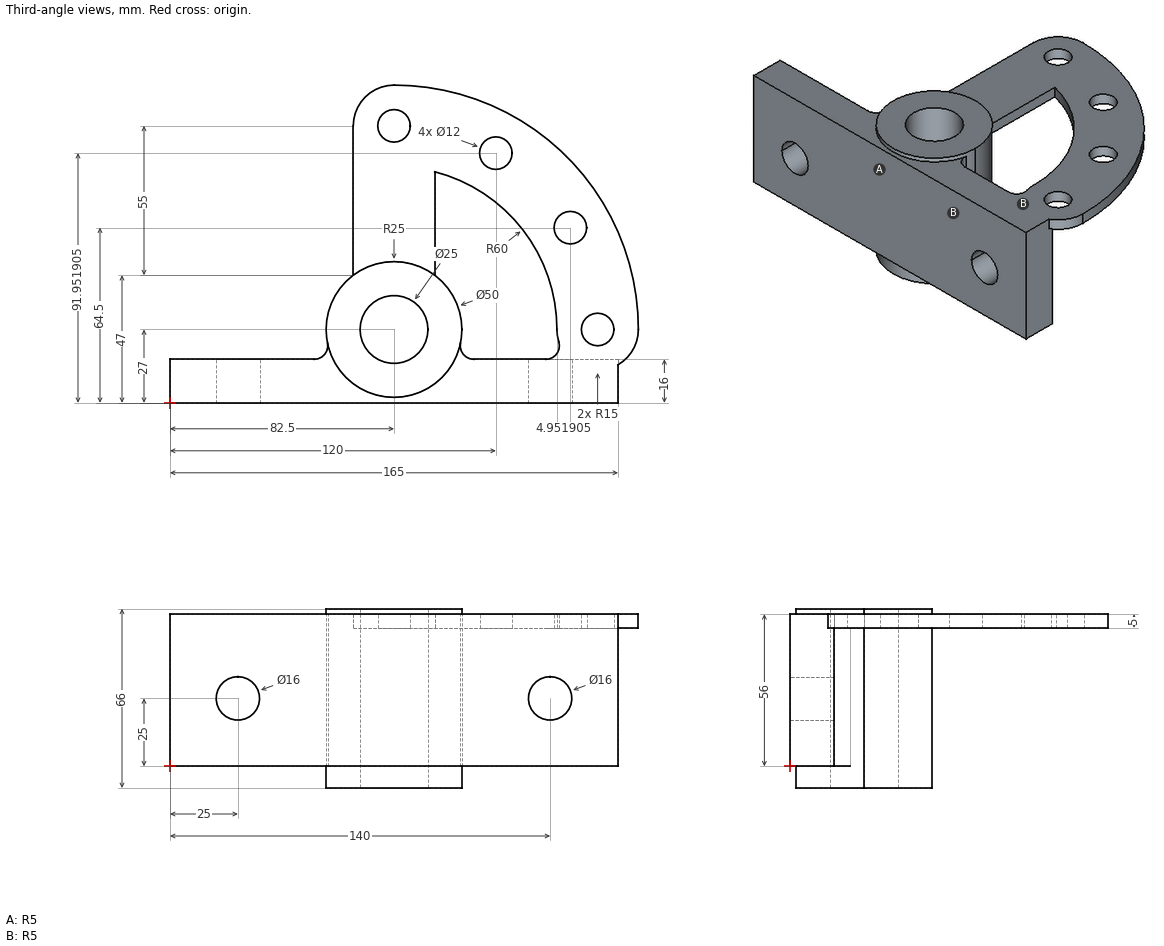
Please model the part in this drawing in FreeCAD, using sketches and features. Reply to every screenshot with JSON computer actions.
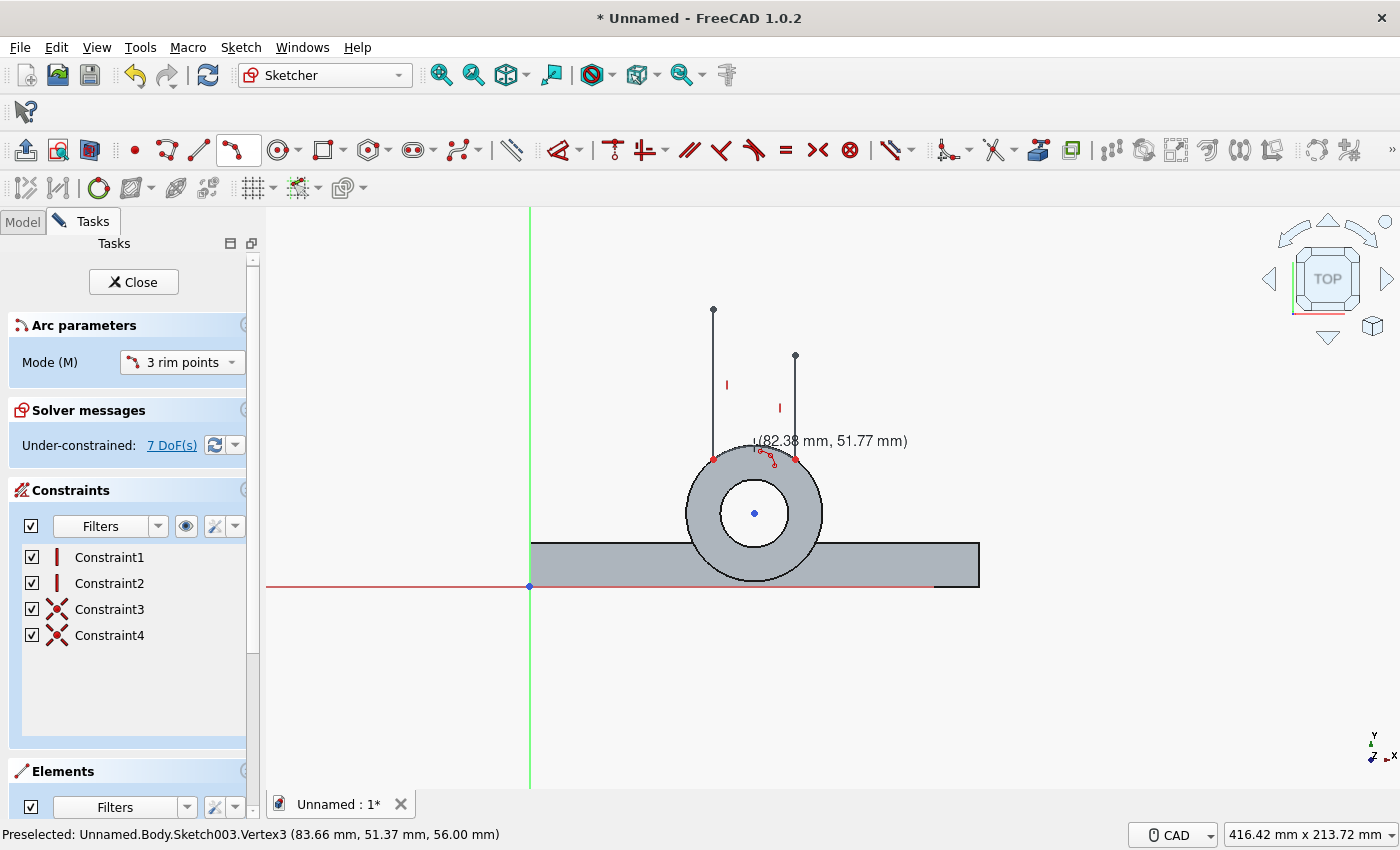
{"action": "left_click", "coordinate": [795, 356]}
{"action": "left_click", "coordinate": [918, 513]}
{"action": "left_click", "coordinate": [884, 413]}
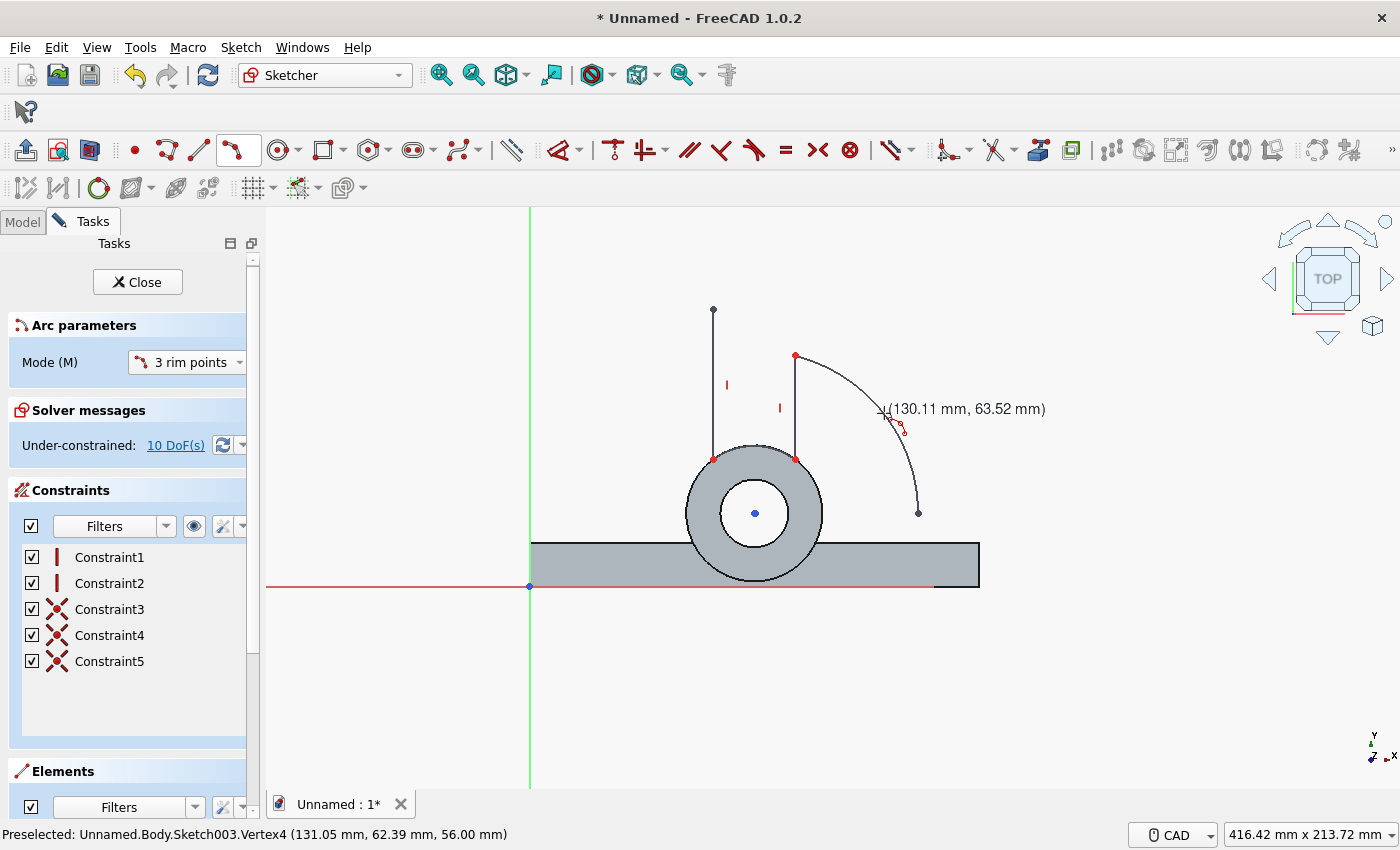
{"action": "left_click", "coordinate": [918, 514]}
{"action": "left_click", "coordinate": [999, 513]}
{"action": "left_click", "coordinate": [959, 554]}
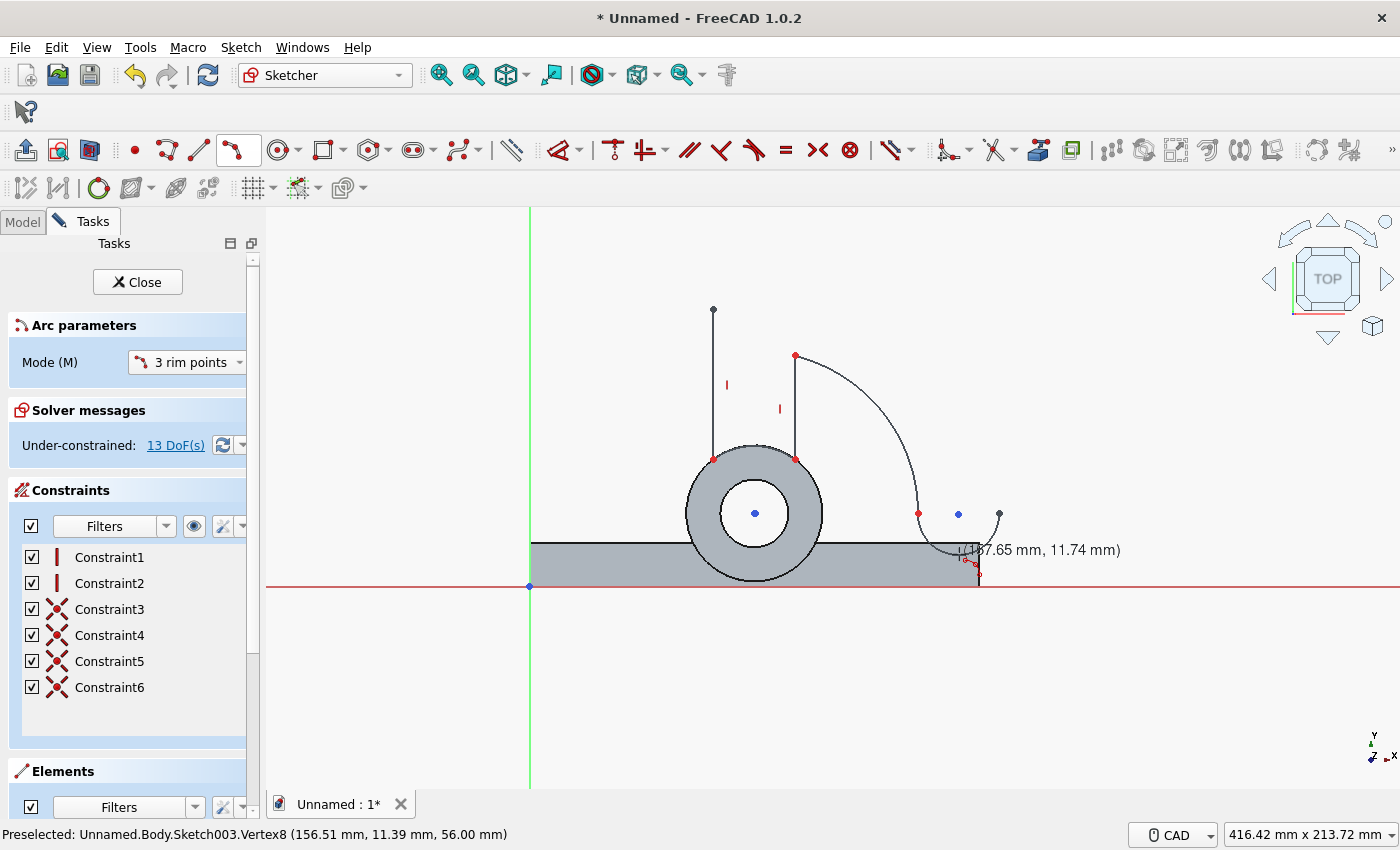
{"action": "left_click", "coordinate": [999, 514]}
{"action": "left_click", "coordinate": [754, 268]}
{"action": "left_click", "coordinate": [928, 340]}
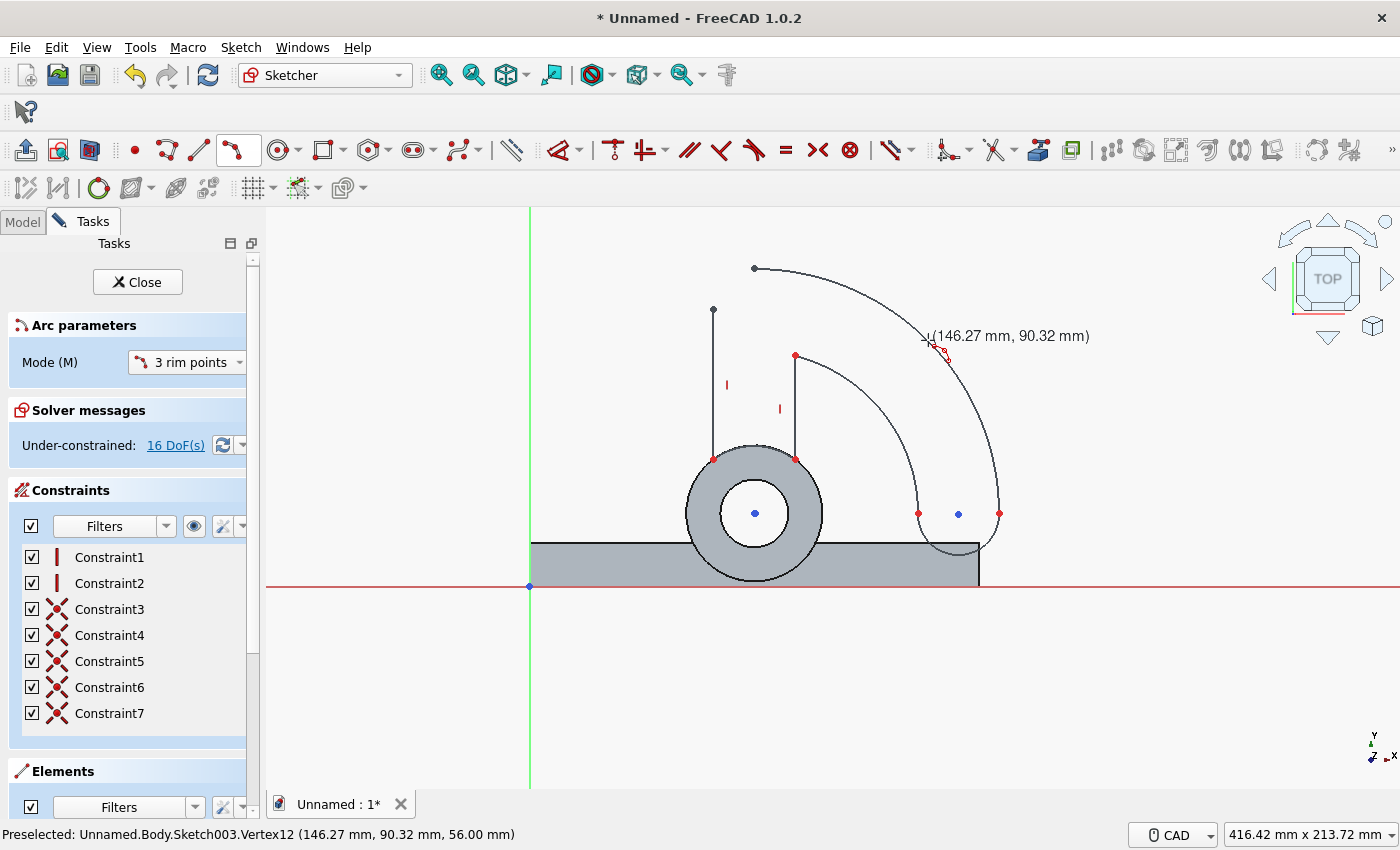
{"action": "left_click", "coordinate": [754, 269]}
{"action": "left_click", "coordinate": [713, 310]}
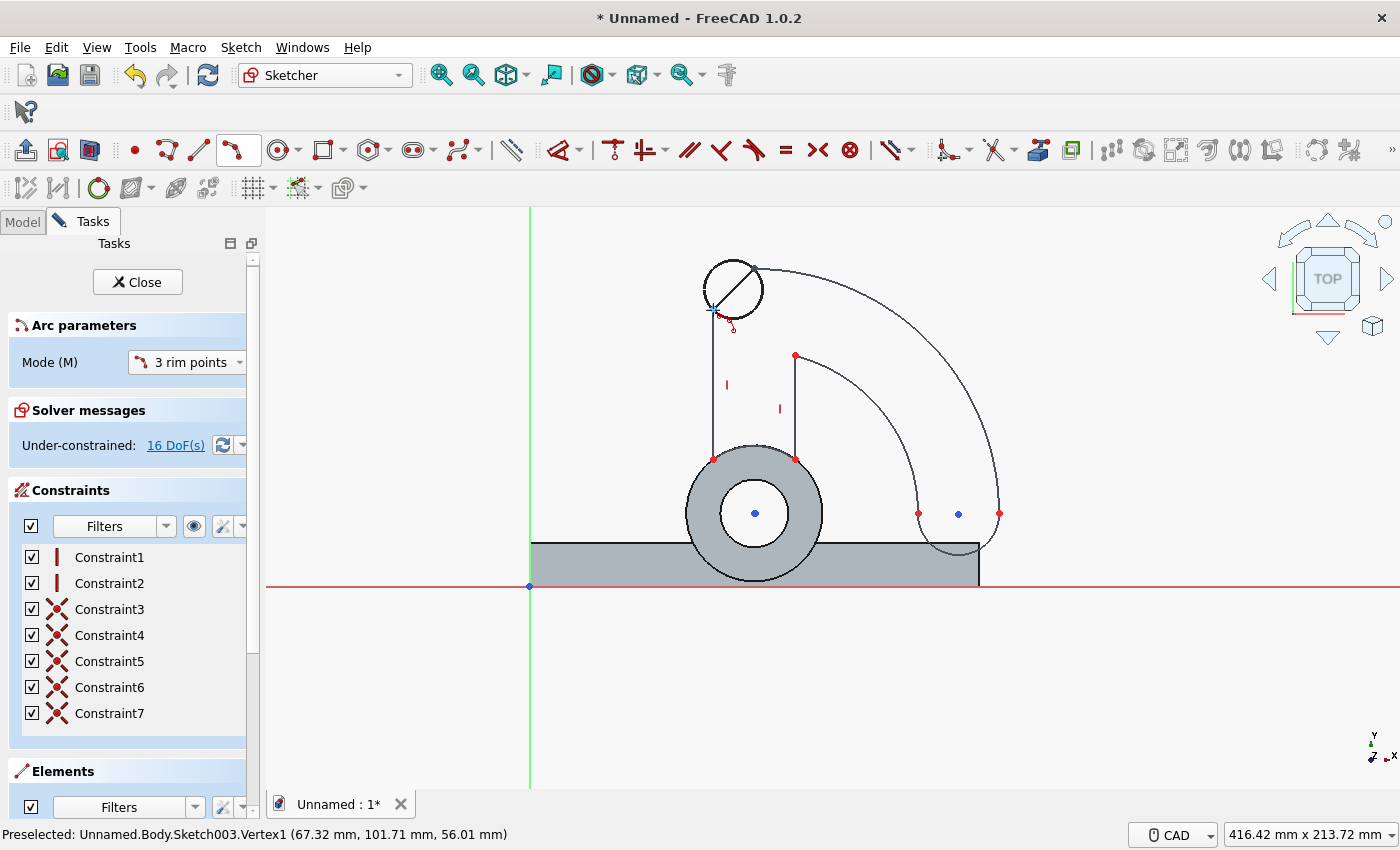
{"action": "scroll", "coordinate": [725, 280], "scroll_direction": "up", "scroll_amount": 2}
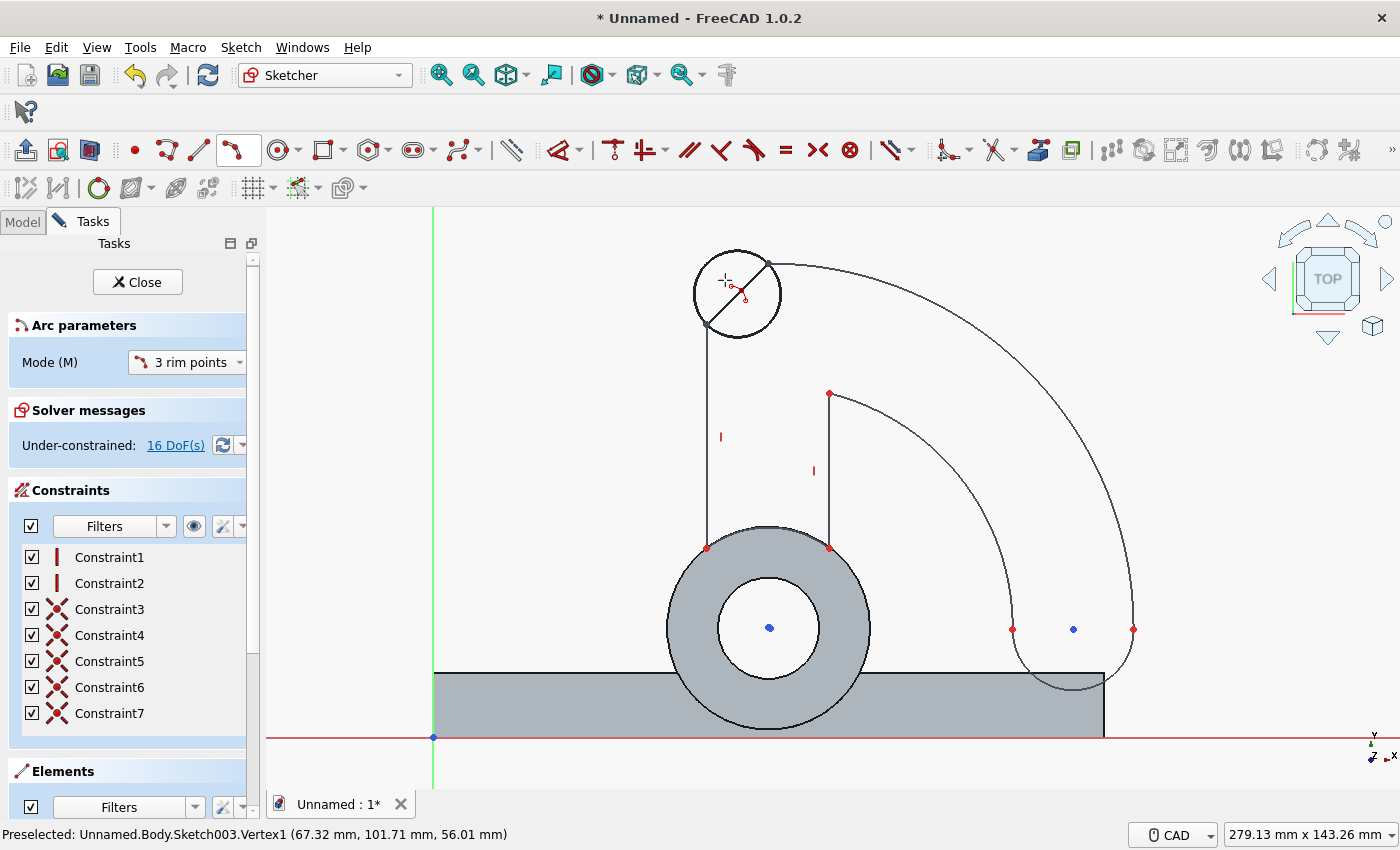
{"action": "left_click", "coordinate": [725, 280]}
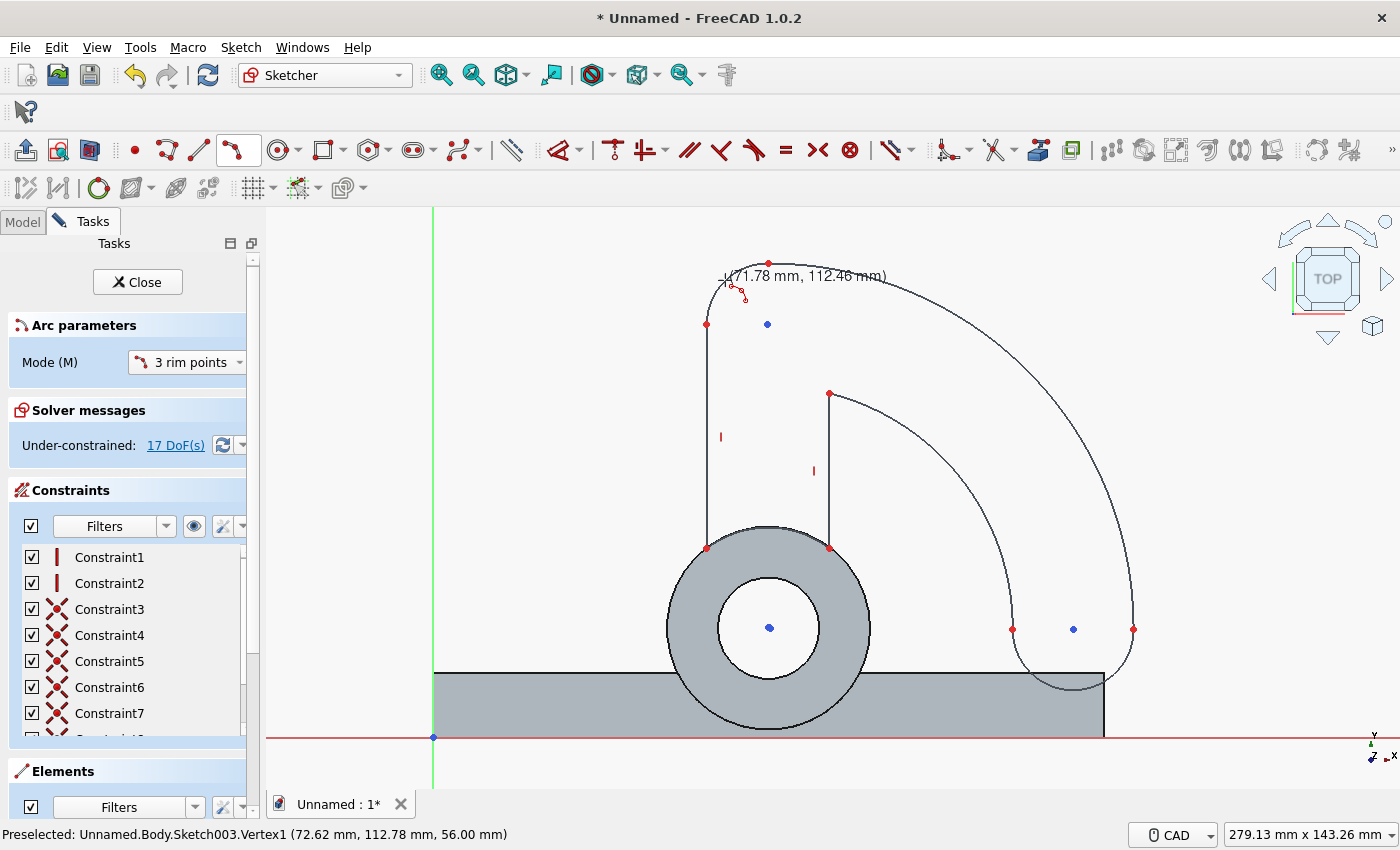
{"action": "key", "text": "g c"}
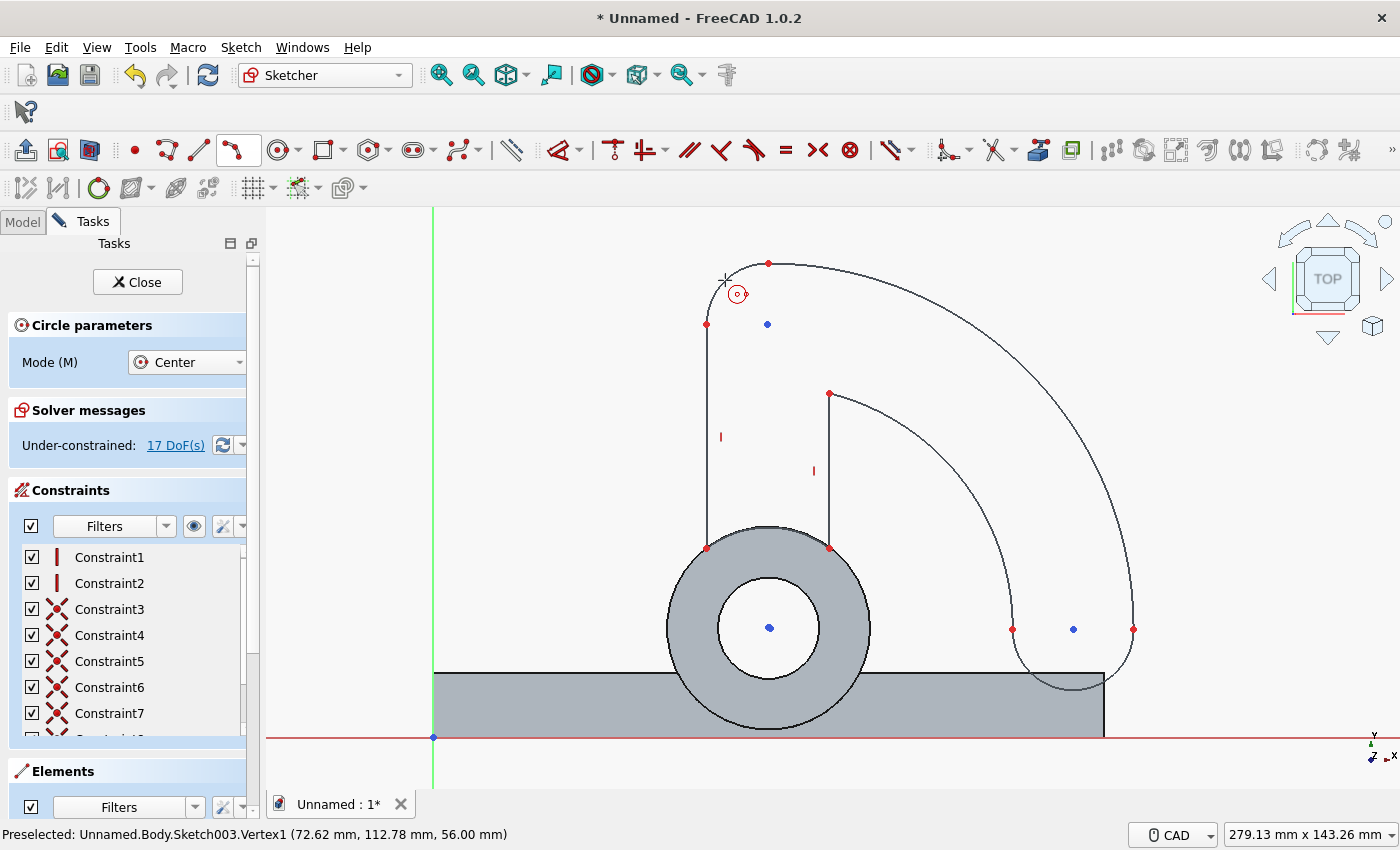
{"action": "left_click", "coordinate": [921, 364]}
{"action": "left_click", "coordinate": [938, 347]}